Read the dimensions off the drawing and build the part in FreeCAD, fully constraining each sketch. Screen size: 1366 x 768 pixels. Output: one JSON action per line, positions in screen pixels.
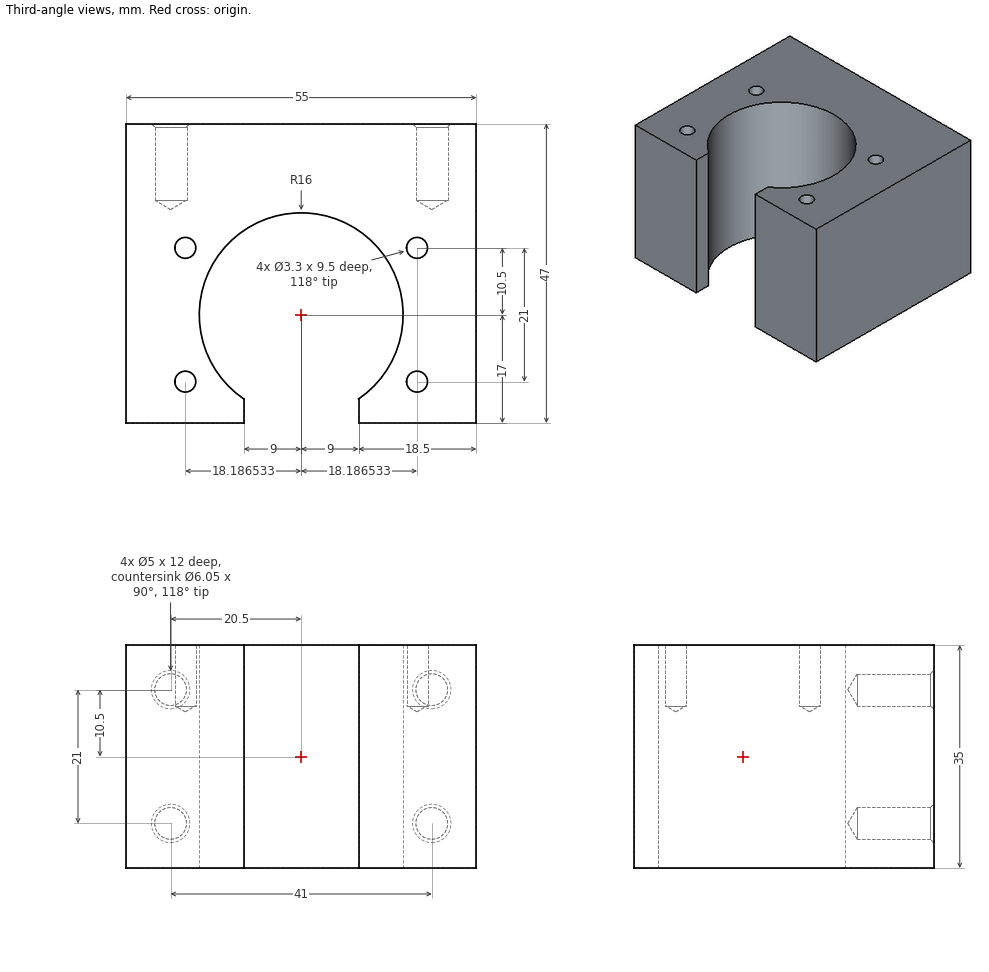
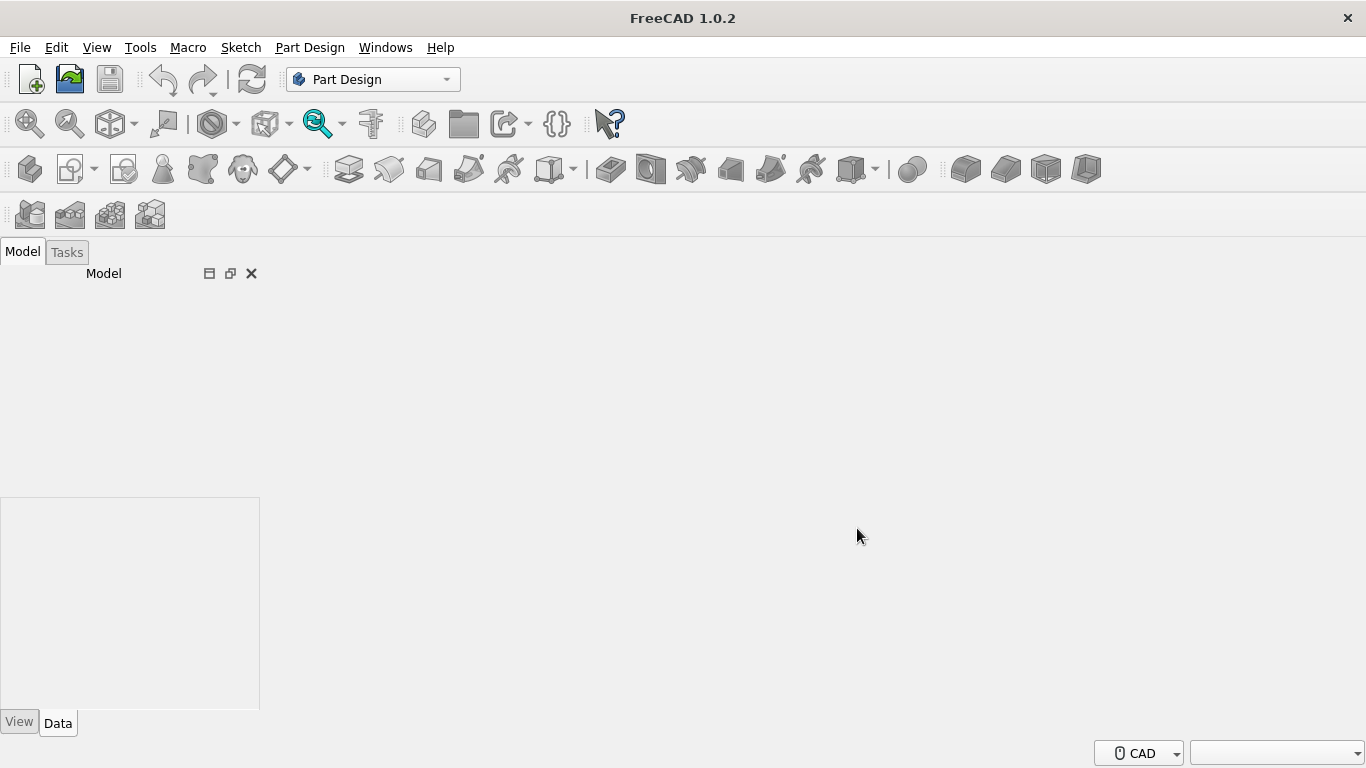
{"action": "left_click", "coordinate": [30, 80]}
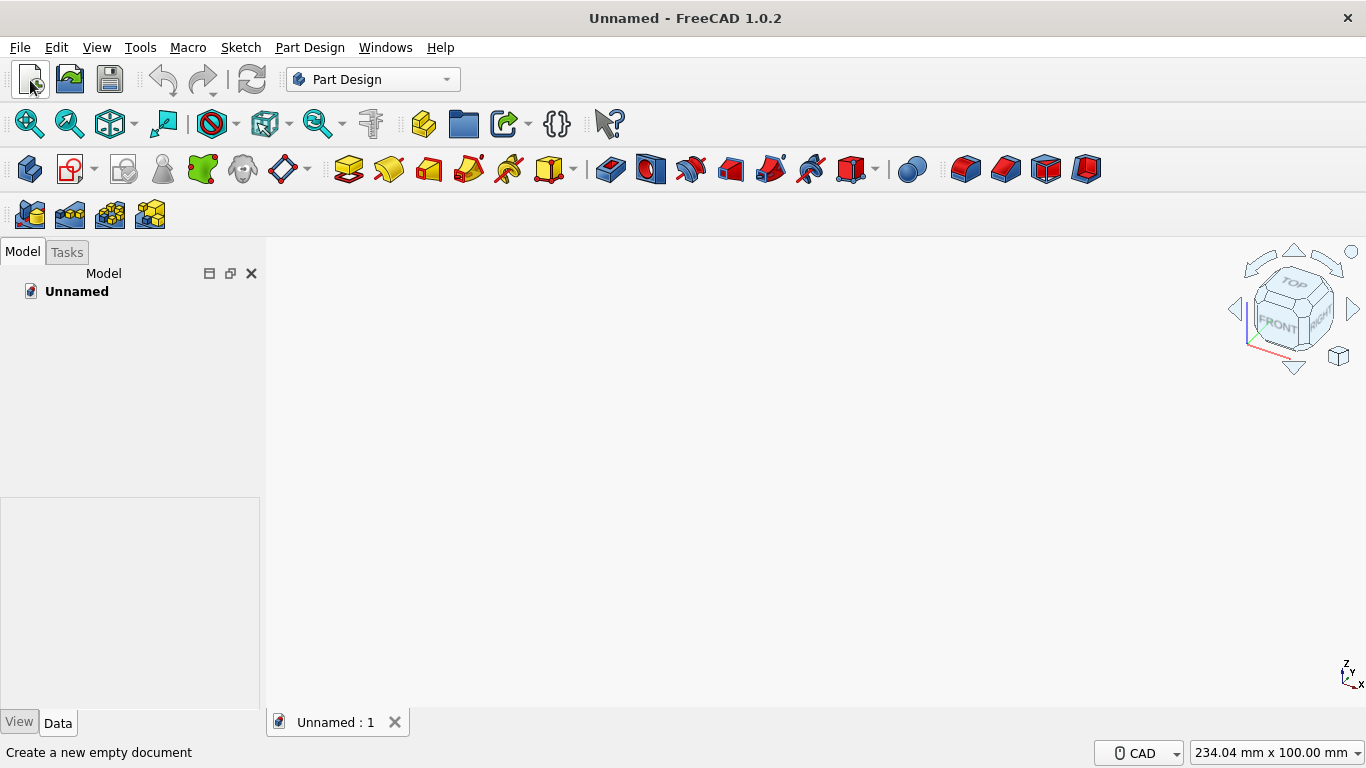
{"action": "left_click", "coordinate": [70, 170]}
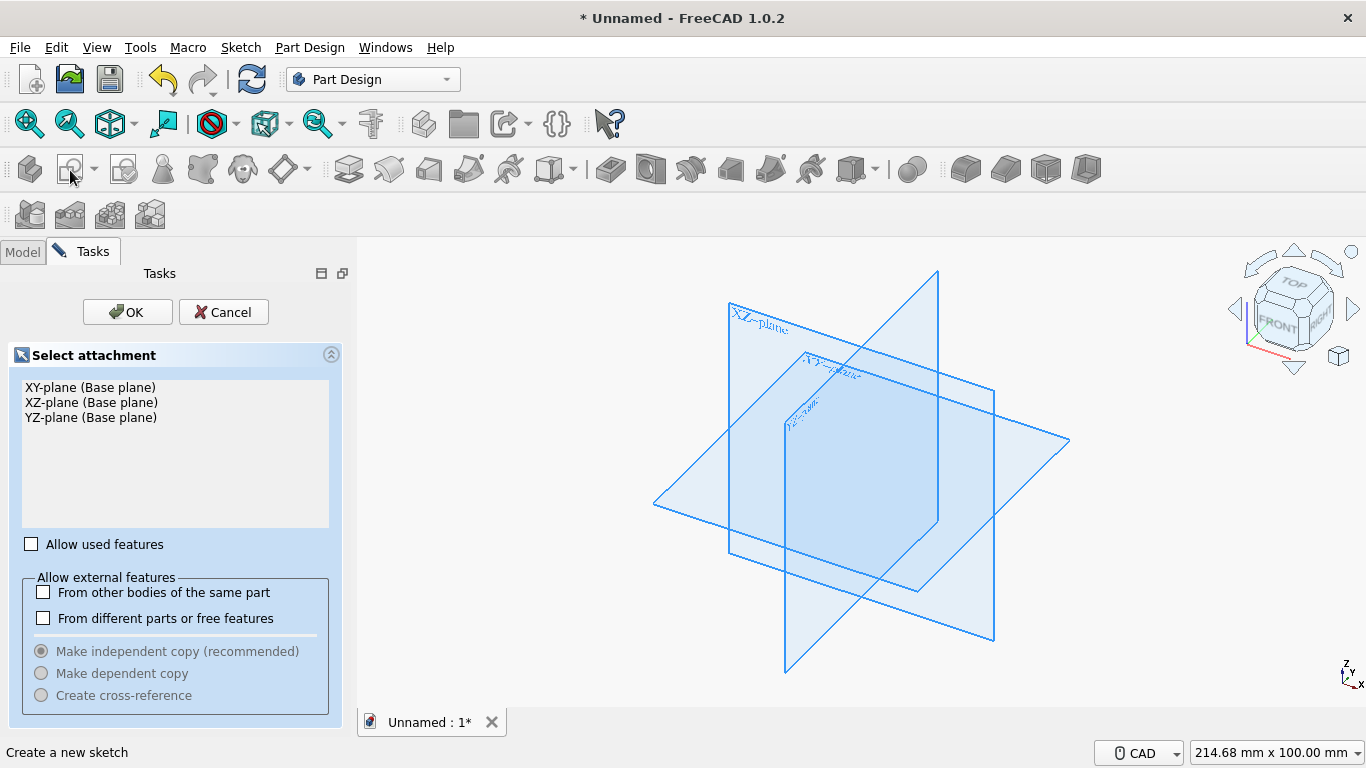
{"action": "left_click", "coordinate": [82, 388]}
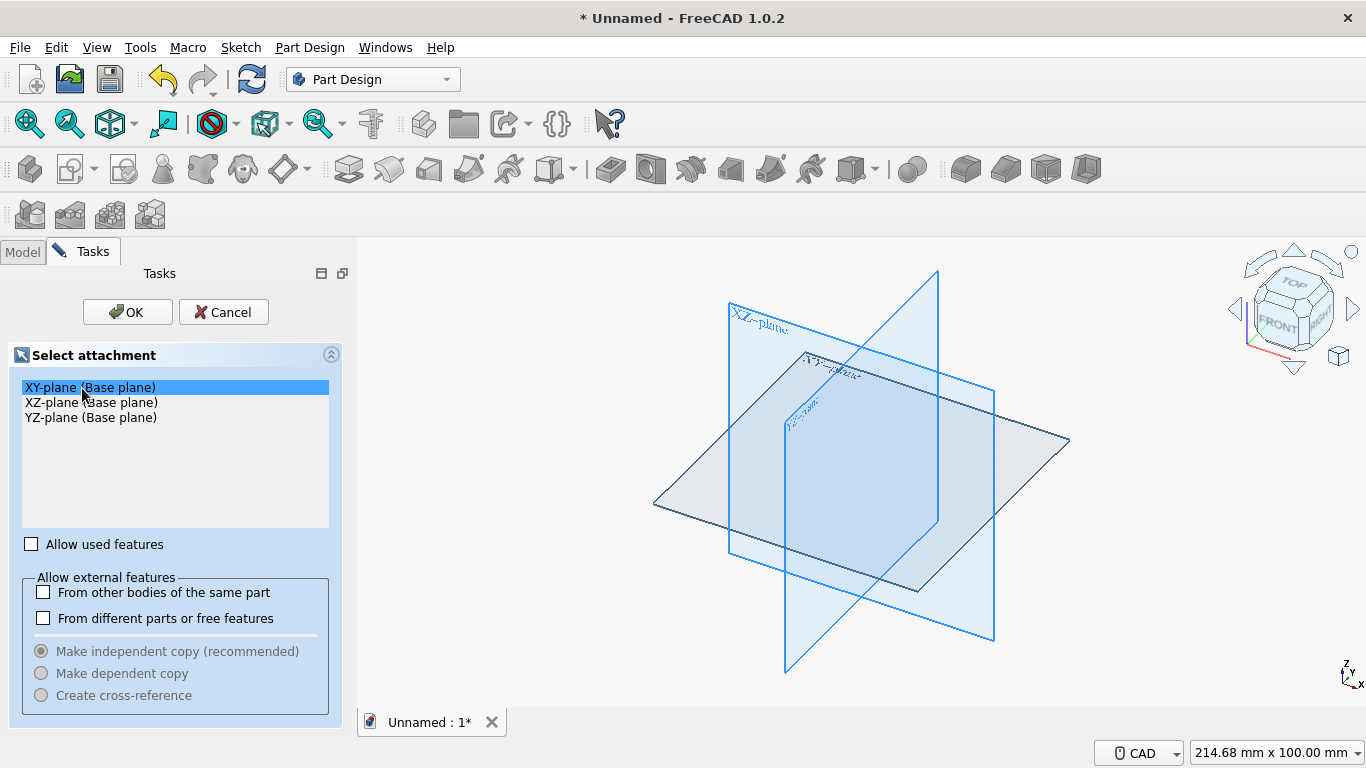
{"action": "left_click", "coordinate": [128, 312]}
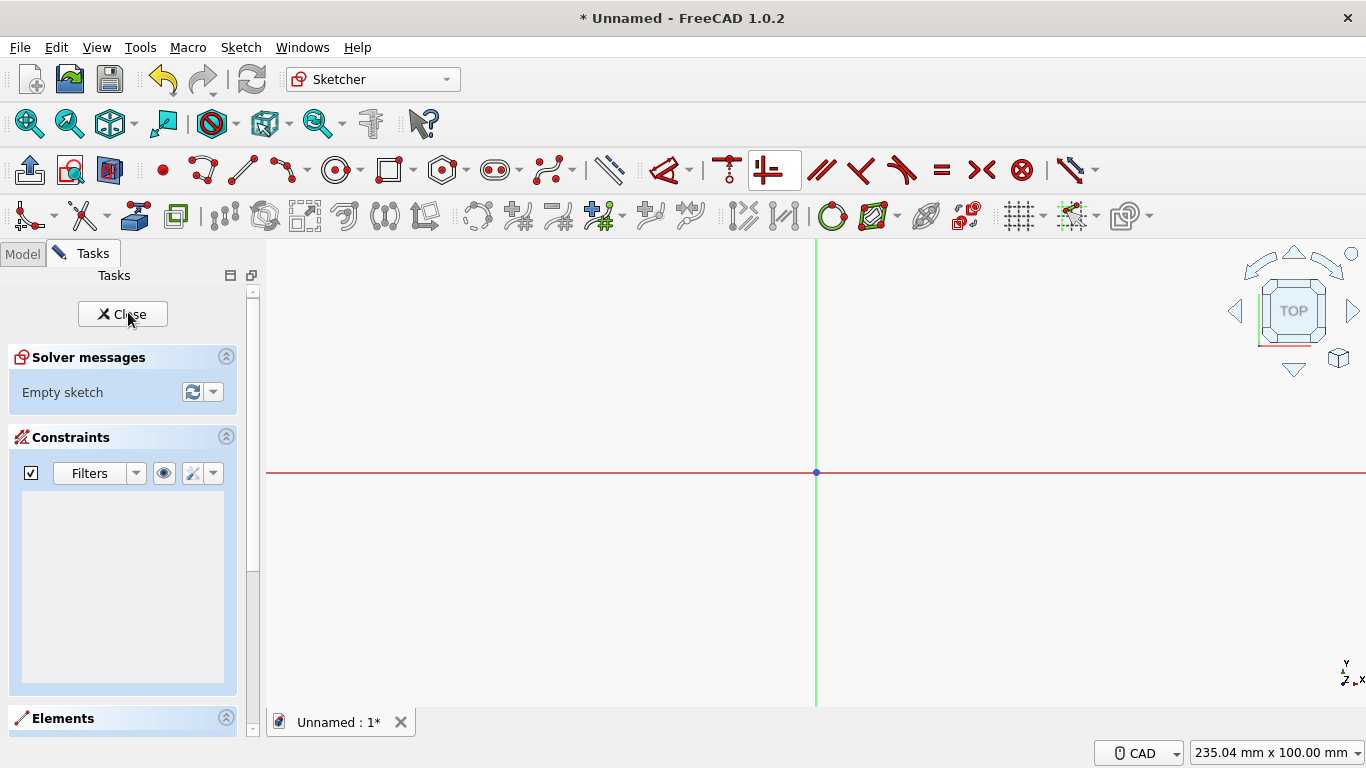
{"action": "left_click", "coordinate": [204, 170]}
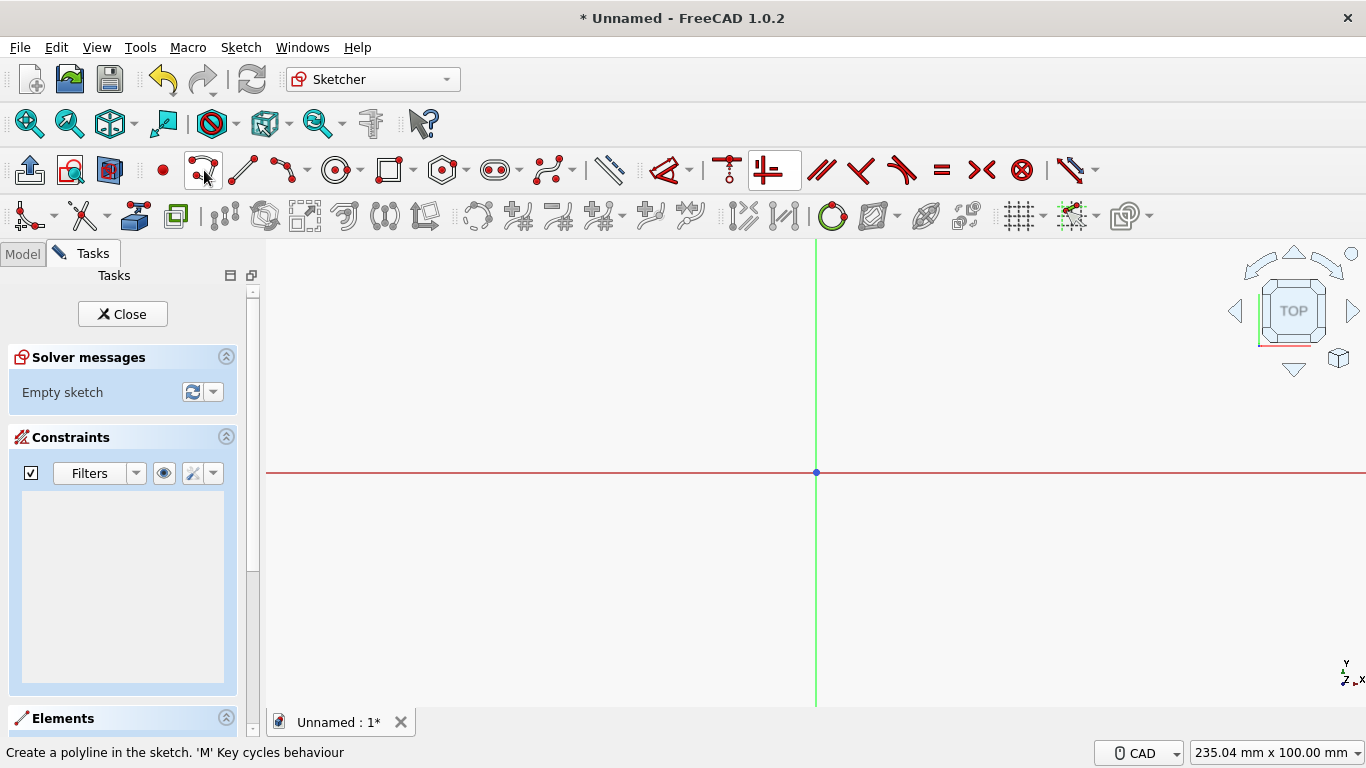
{"action": "left_click", "coordinate": [858, 535]}
{"action": "left_click", "coordinate": [858, 553]}
{"action": "left_click", "coordinate": [945, 553]}
{"action": "left_click", "coordinate": [945, 333]}
{"action": "left_click", "coordinate": [687, 333]}
{"action": "left_click", "coordinate": [687, 553]}
{"action": "left_click", "coordinate": [774, 553]}
{"action": "left_click", "coordinate": [774, 535]}
{"action": "right_click", "coordinate": [774, 535]}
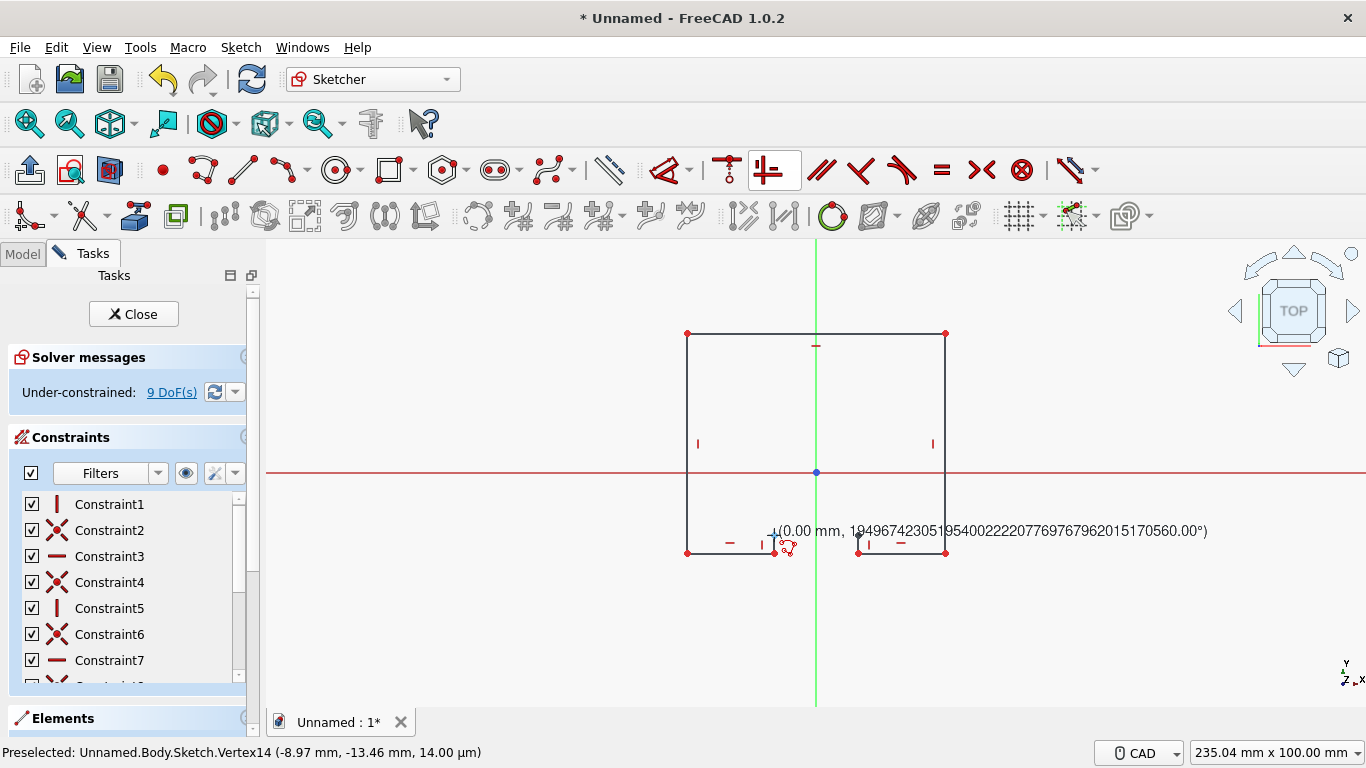
{"action": "left_click", "coordinate": [284, 170]}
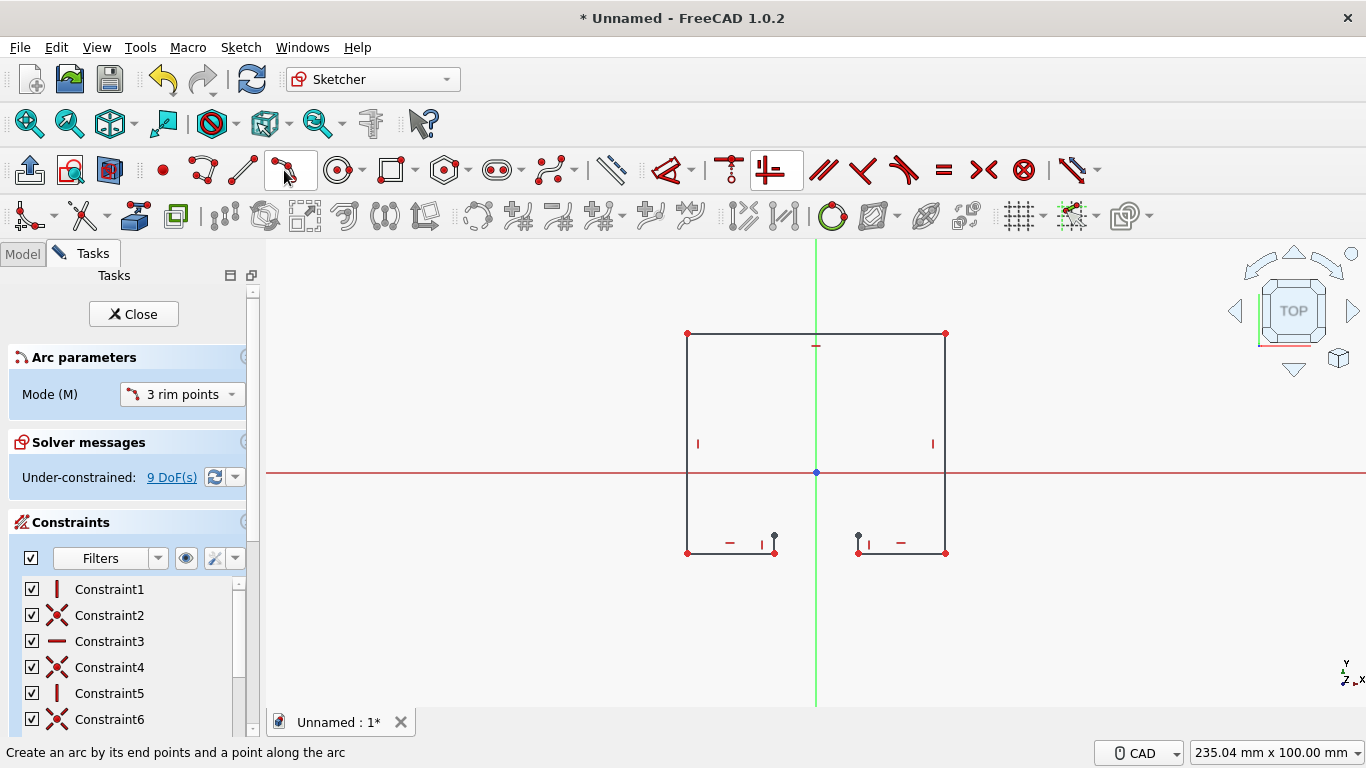
{"action": "scroll", "coordinate": [774, 535], "scroll_direction": "up", "scroll_amount": 3}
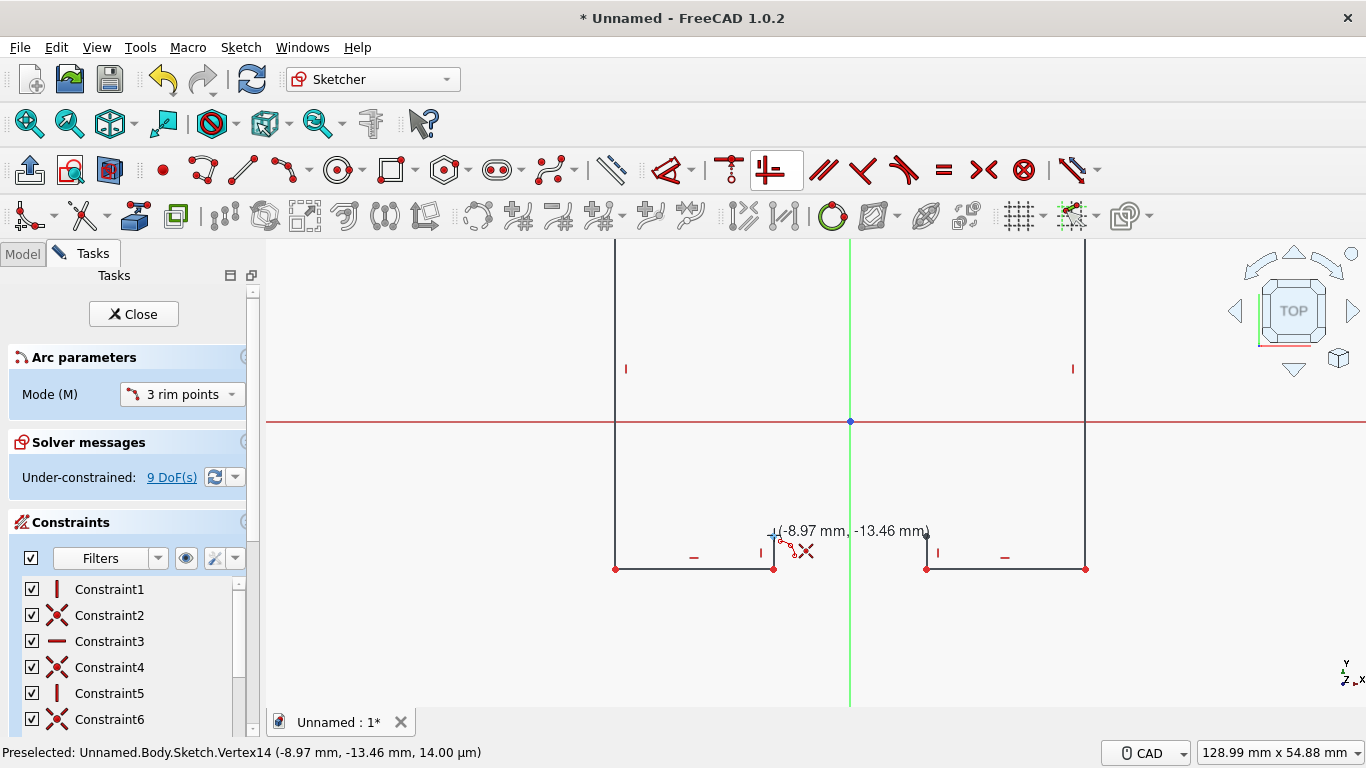
{"action": "left_click", "coordinate": [774, 536]}
{"action": "left_click", "coordinate": [927, 536]}
{"action": "left_click", "coordinate": [917, 302]}
{"action": "key", "text": "Escape"}